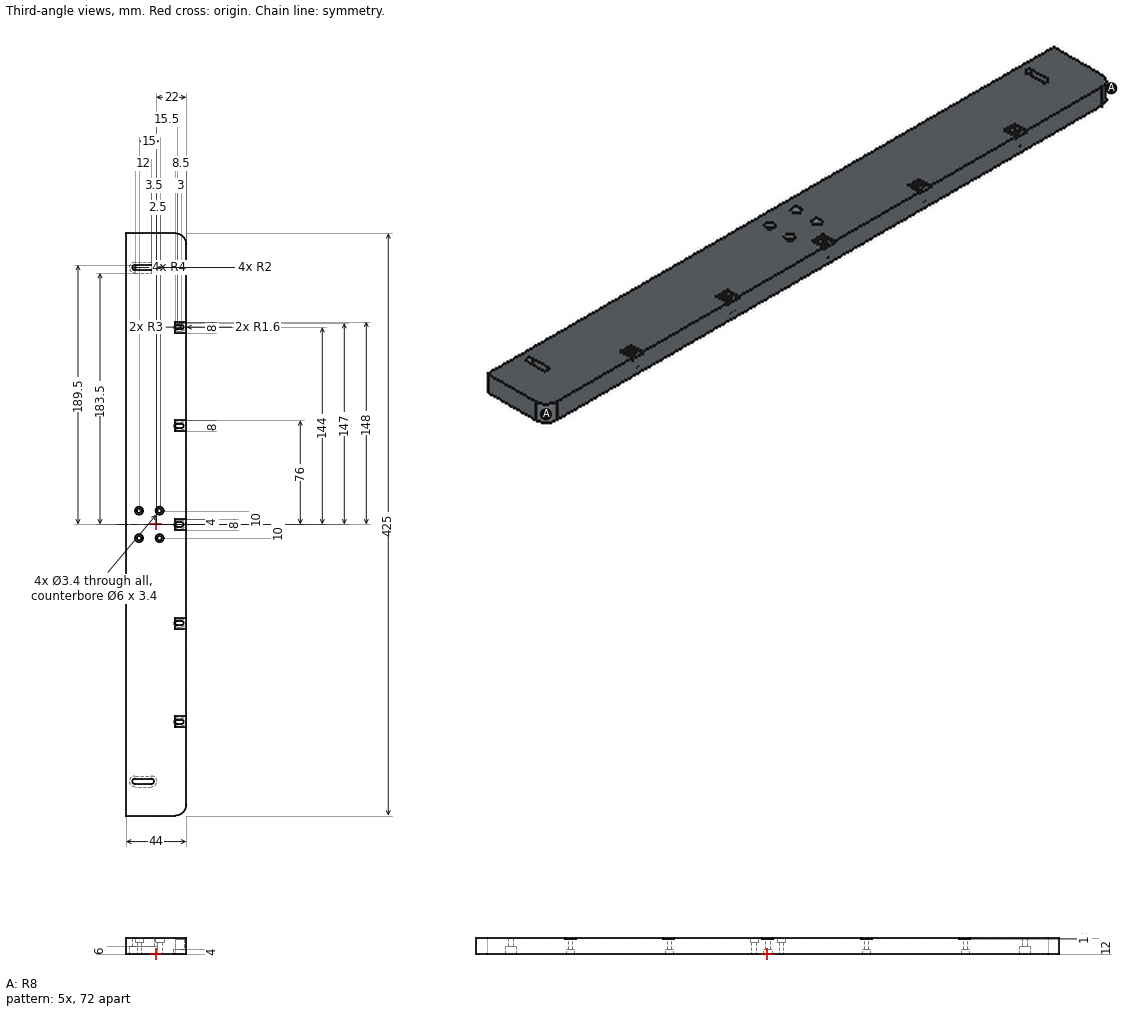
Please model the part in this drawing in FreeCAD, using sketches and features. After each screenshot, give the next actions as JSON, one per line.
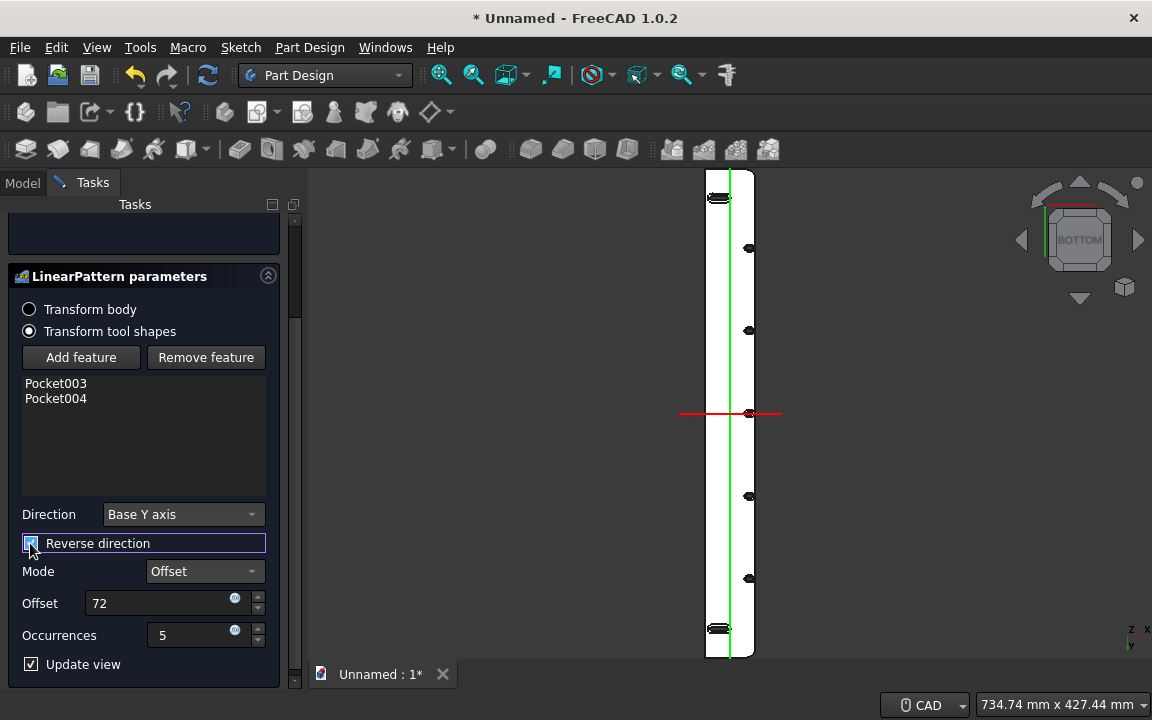
{"action": "scroll", "coordinate": [295, 451], "scroll_direction": "up", "scroll_amount": 3}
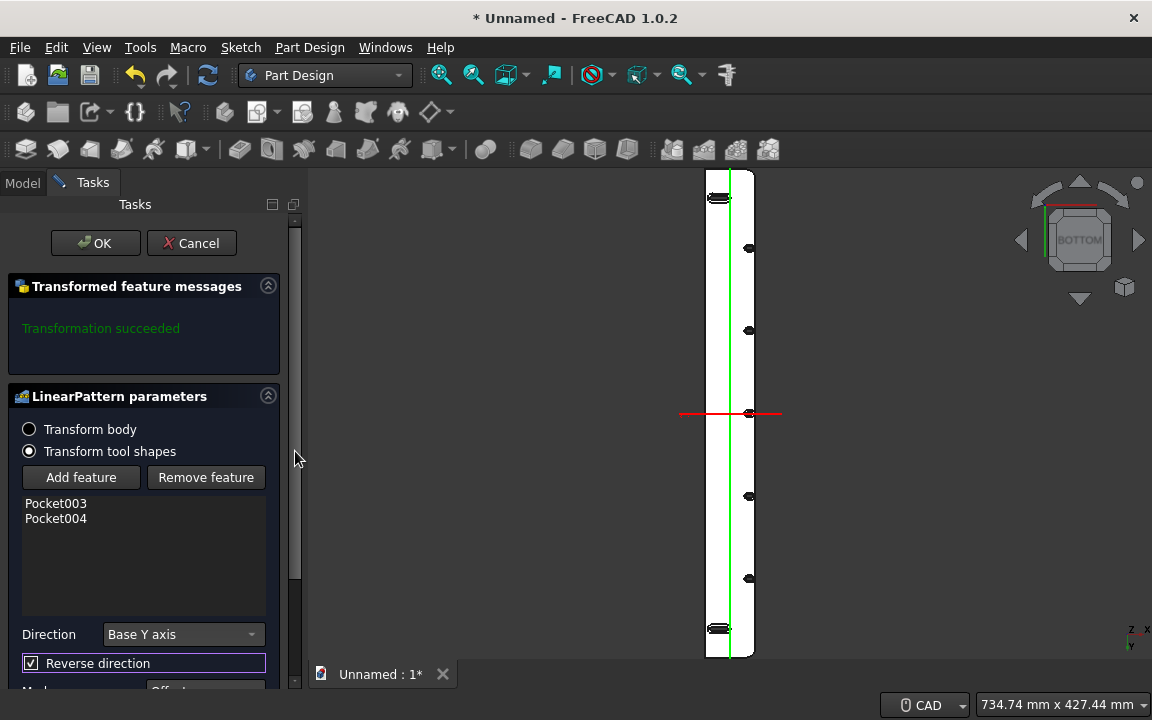
{"action": "left_click", "coordinate": [96, 243]}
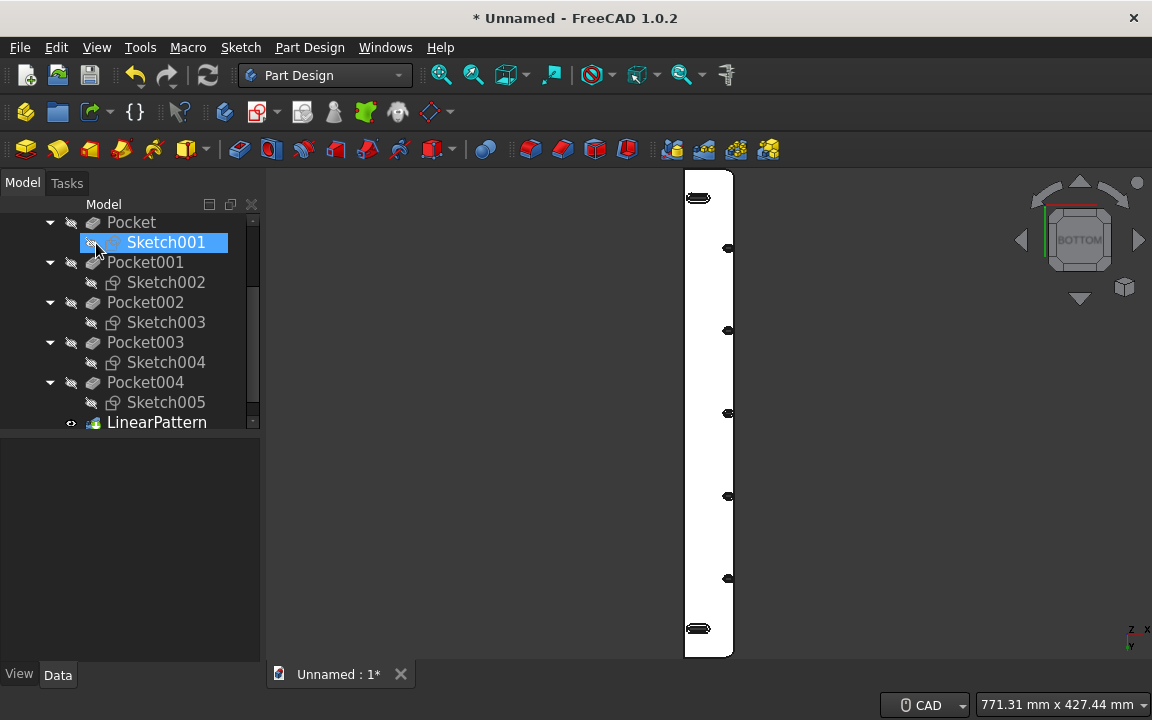
{"action": "key", "text": "0"}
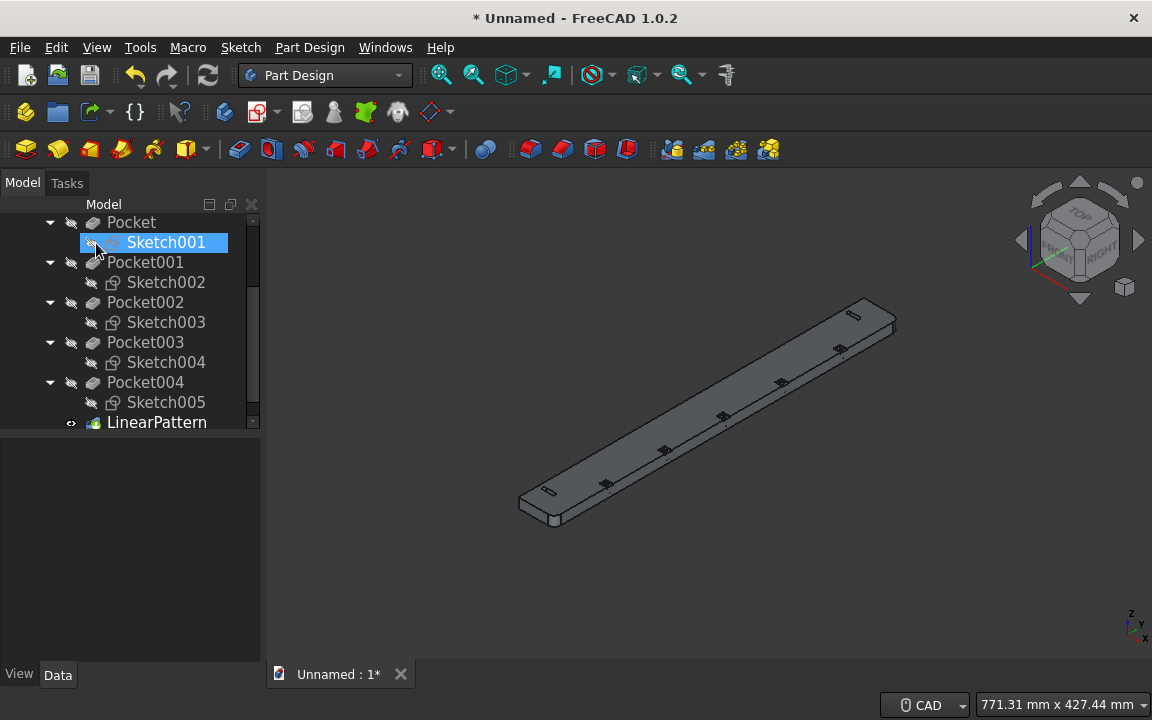
{"action": "left_click", "coordinate": [808, 350]}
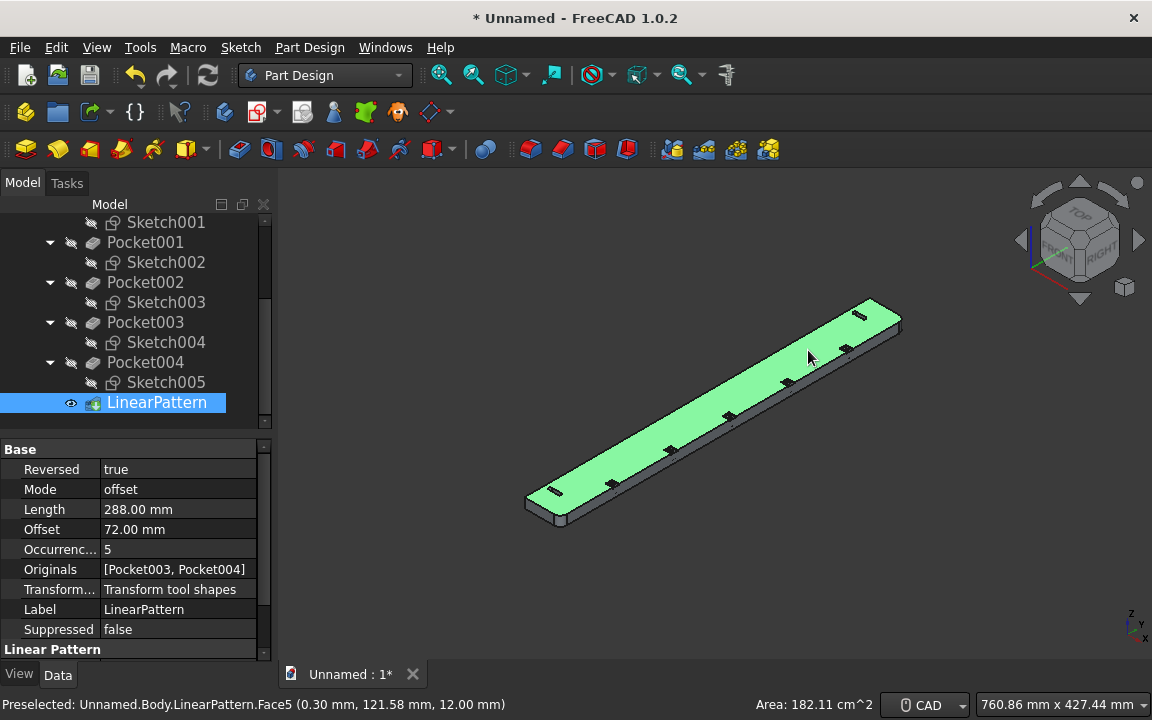
{"action": "left_click", "coordinate": [258, 112]}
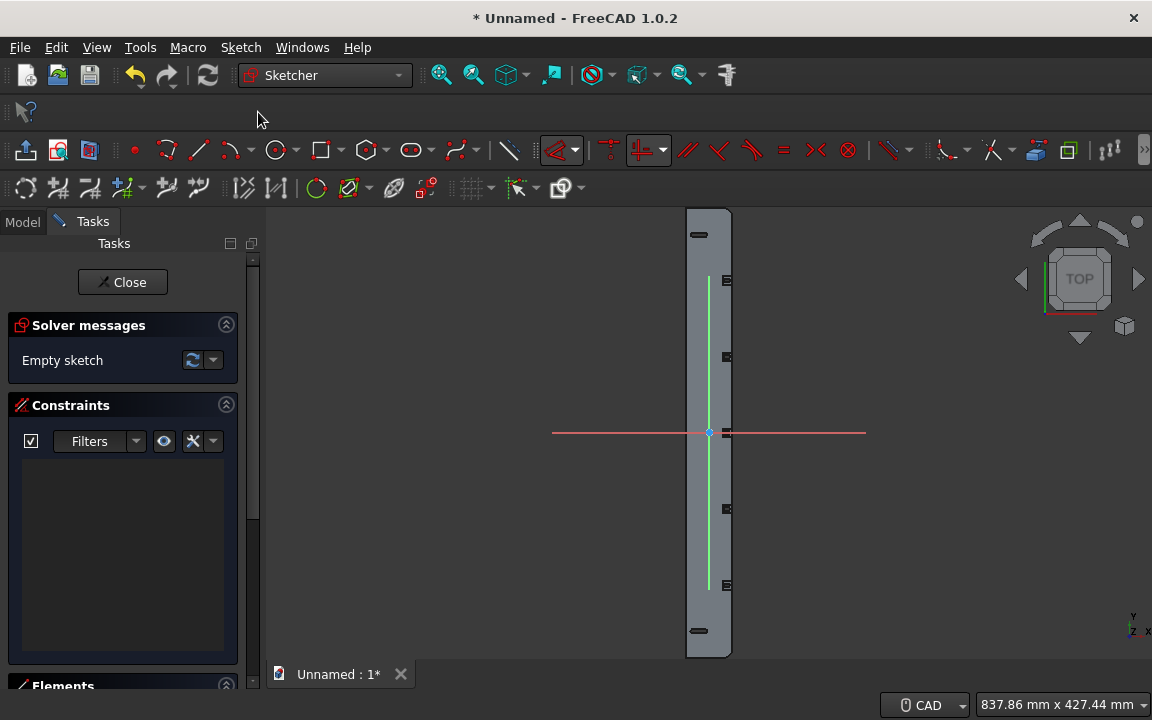
{"action": "scroll", "coordinate": [710, 433], "scroll_direction": "up", "scroll_amount": 12}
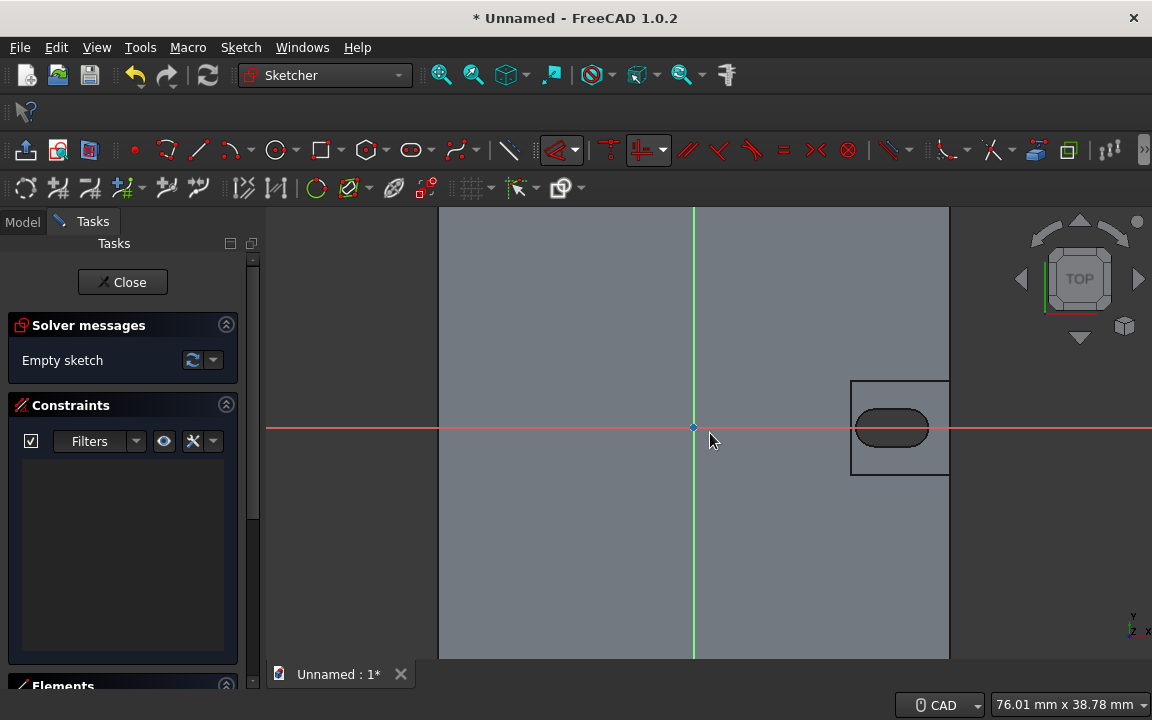
{"action": "key", "text": "g c"}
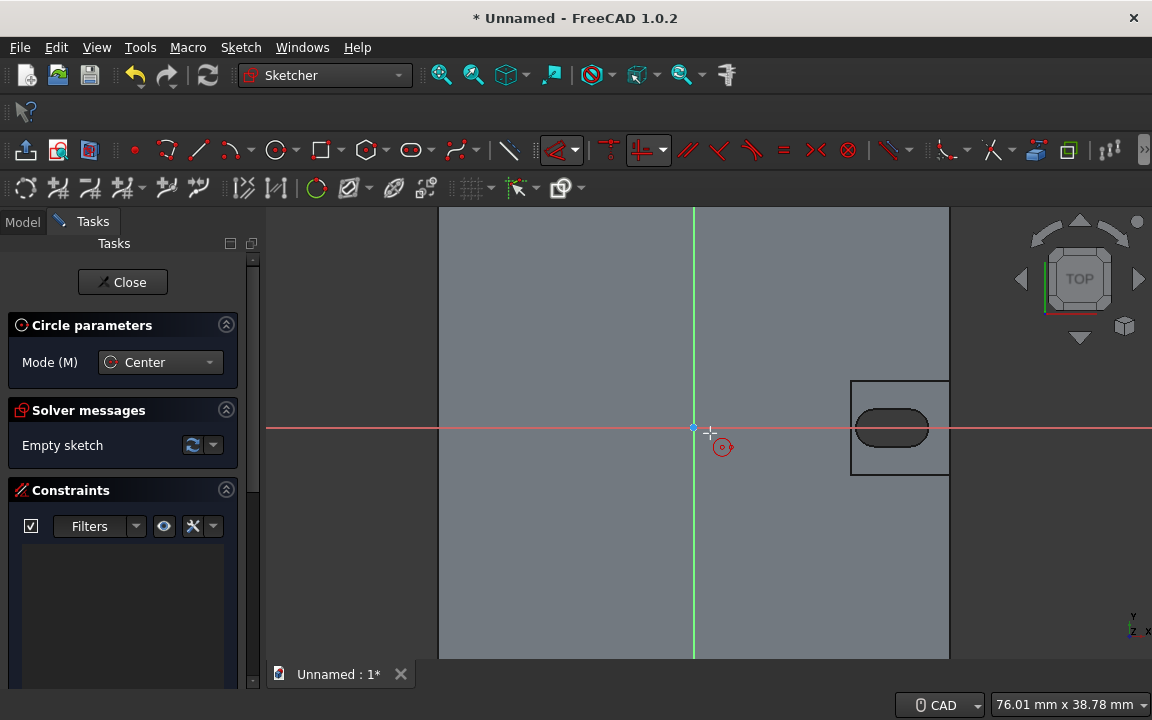
{"action": "left_click", "coordinate": [723, 311]}
{"action": "left_click", "coordinate": [737, 297]}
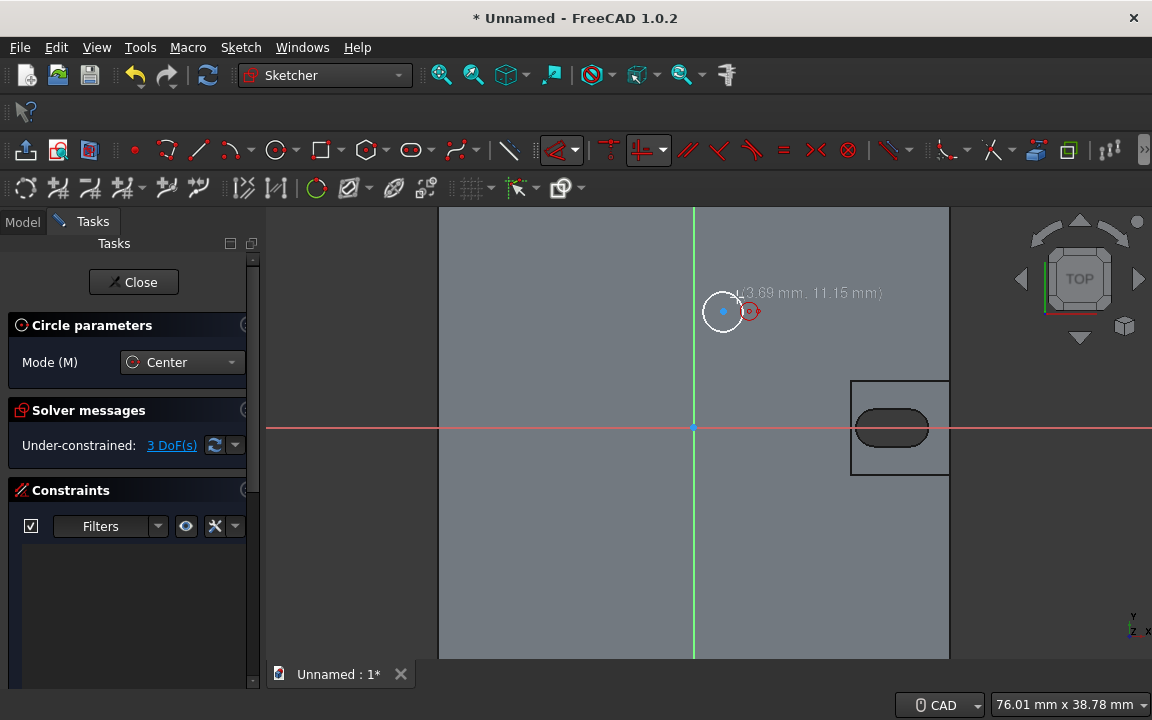
{"action": "left_click", "coordinate": [548, 311]}
{"action": "left_click", "coordinate": [562, 297]}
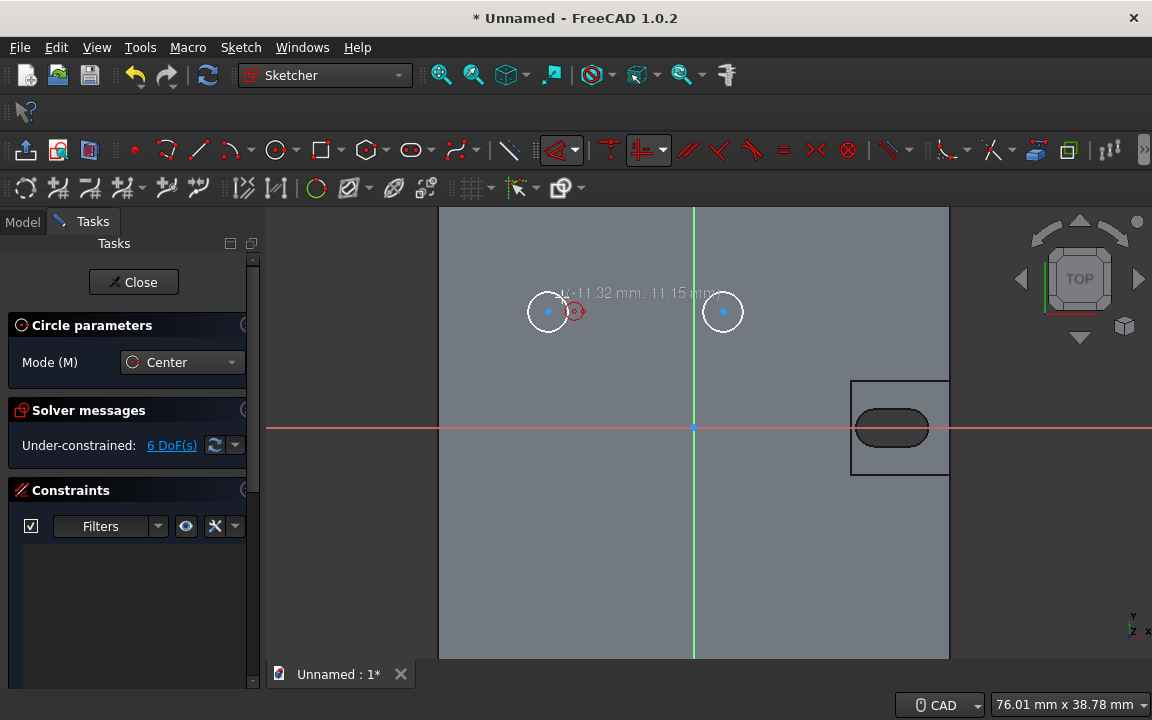
{"action": "left_click", "coordinate": [723, 545]}
{"action": "left_click", "coordinate": [737, 531]}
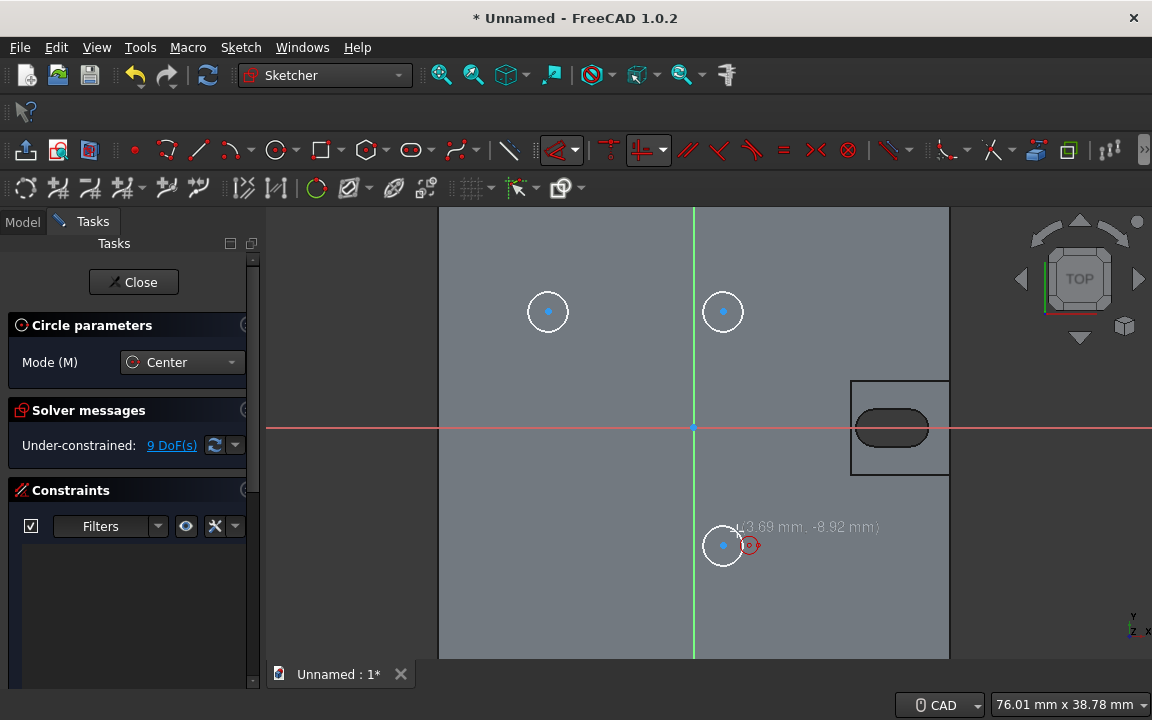
{"action": "left_click", "coordinate": [548, 545]}
{"action": "left_click", "coordinate": [562, 531]}
{"action": "key", "text": "Escape"}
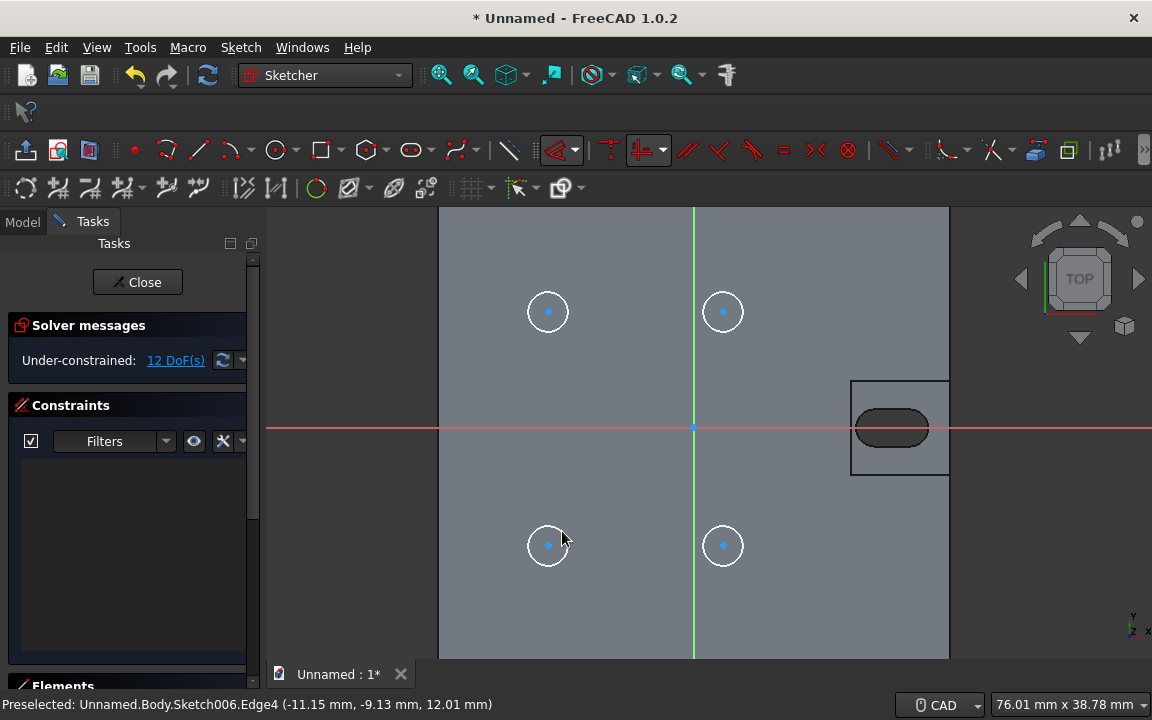
{"action": "left_click", "coordinate": [737, 298]}